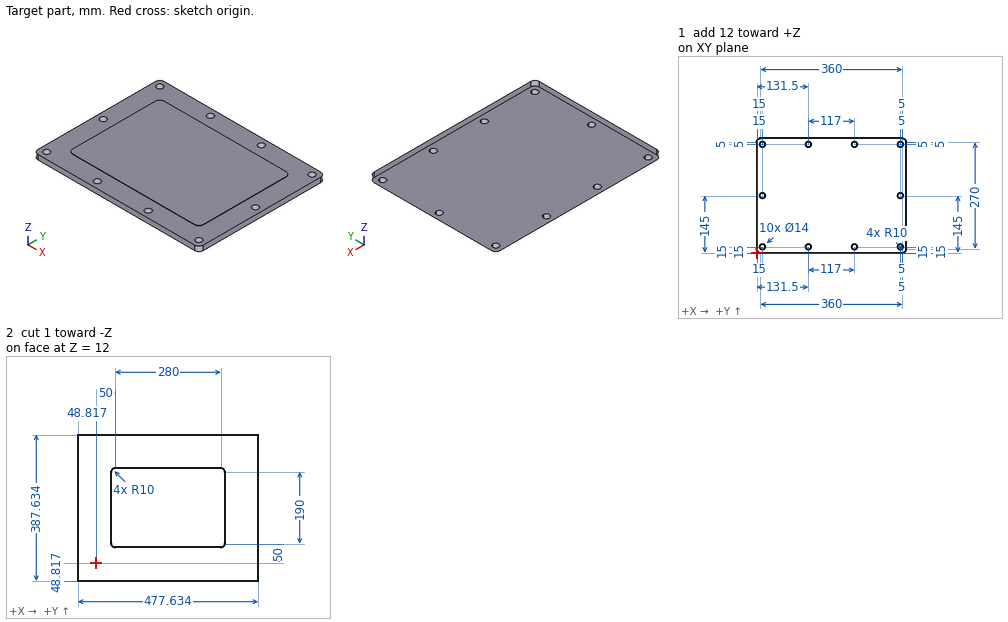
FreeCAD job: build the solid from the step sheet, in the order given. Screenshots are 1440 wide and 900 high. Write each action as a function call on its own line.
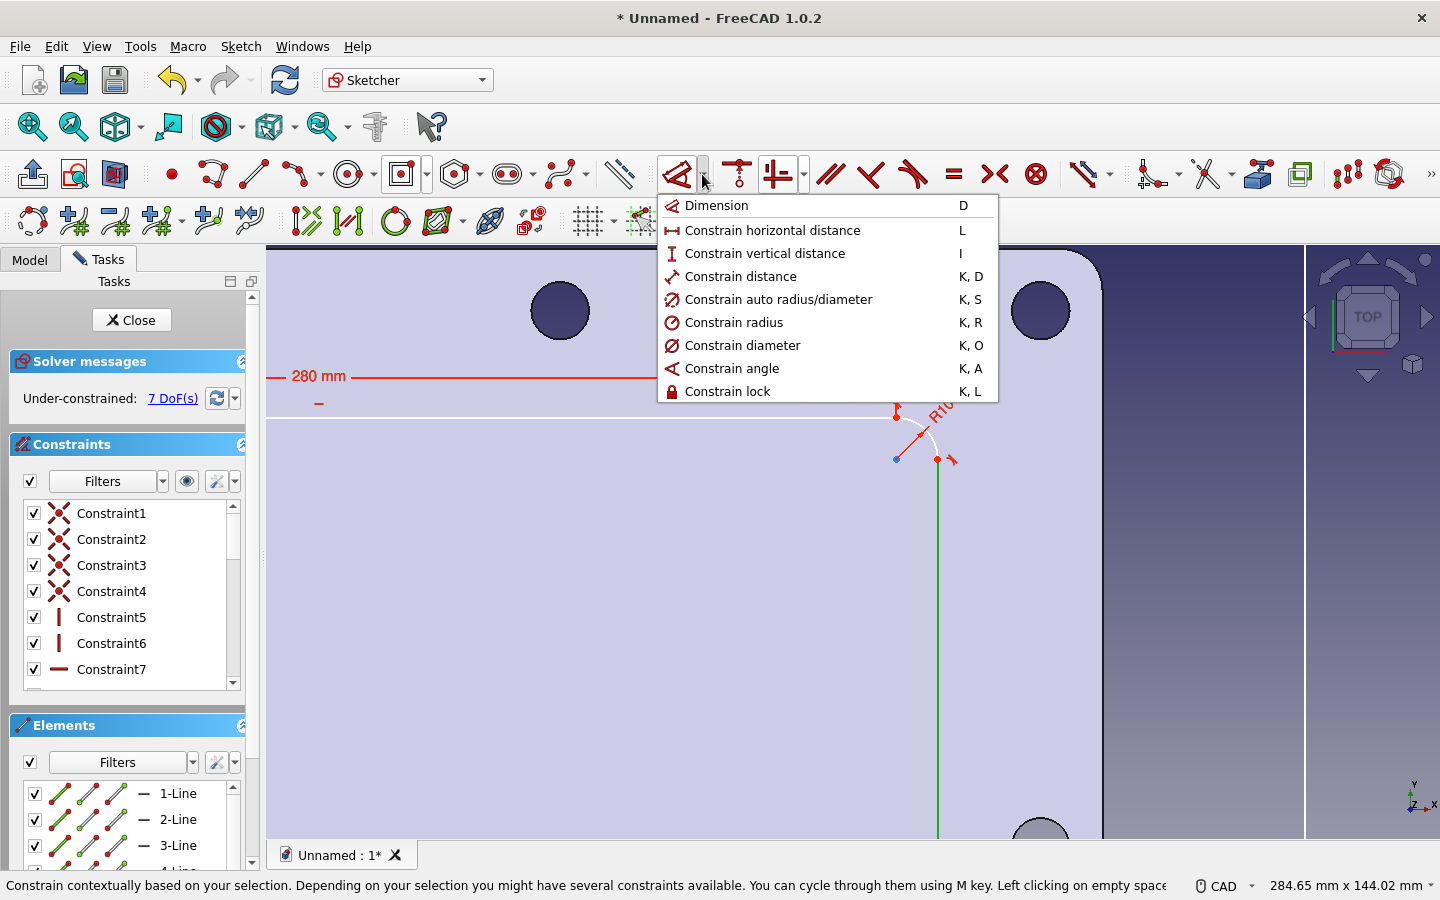
click(828, 254)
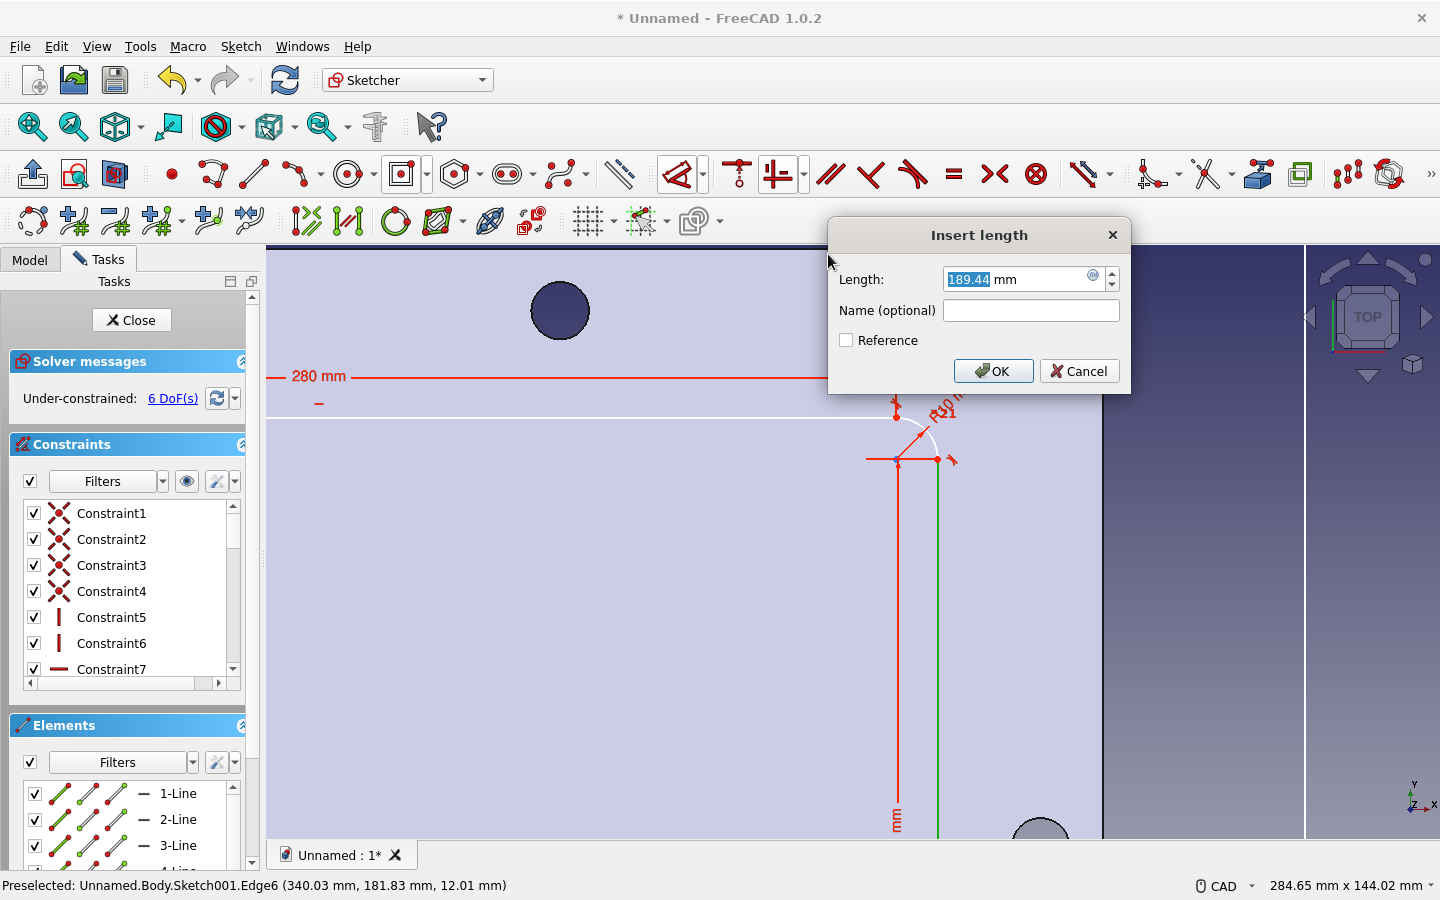
text(190)
key(Return)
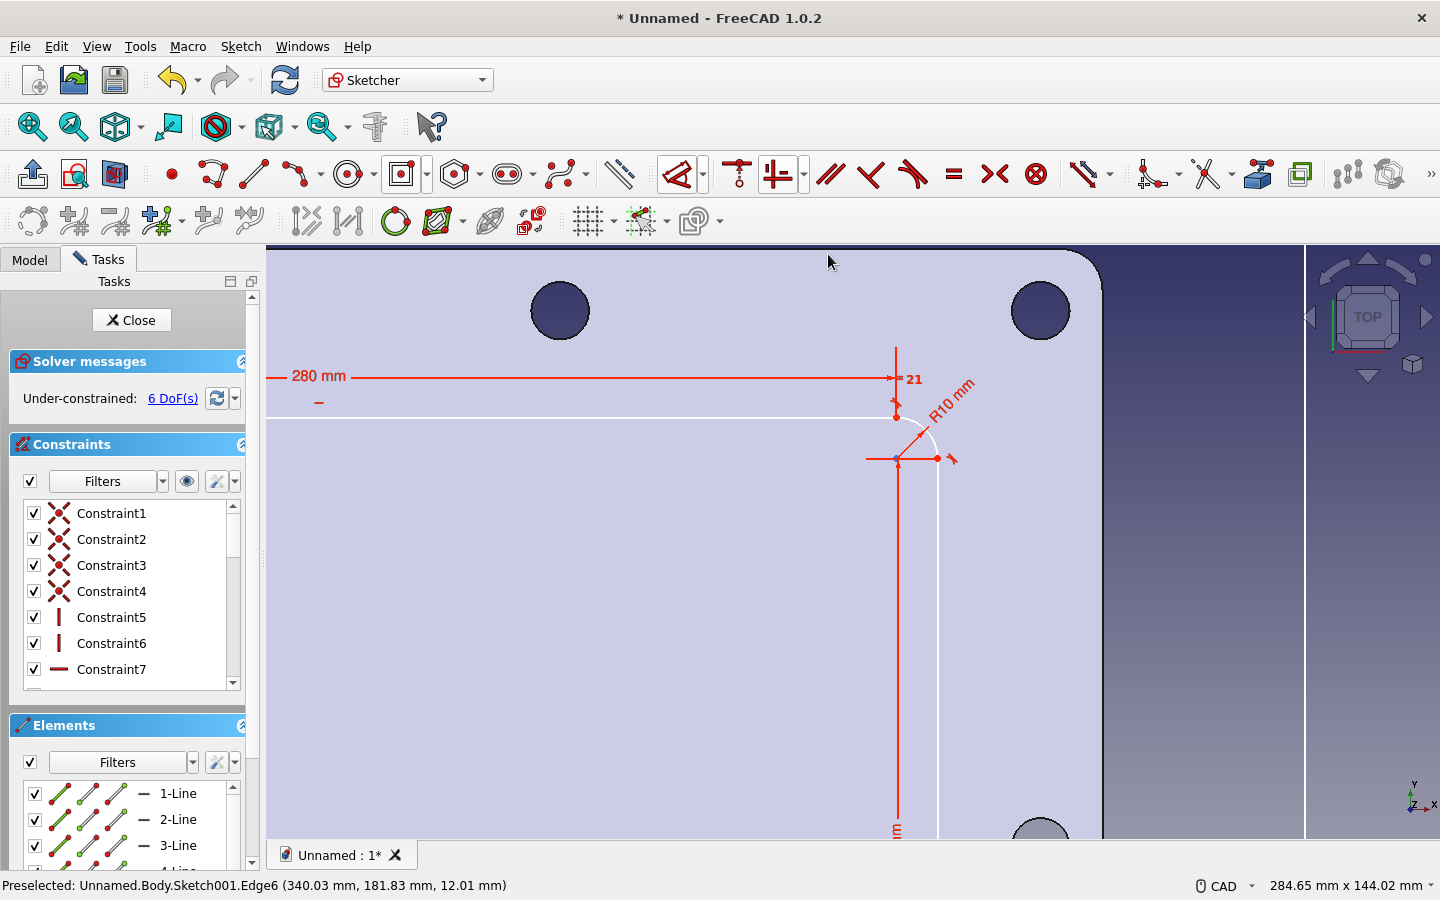
scroll(937, 442, down, 7)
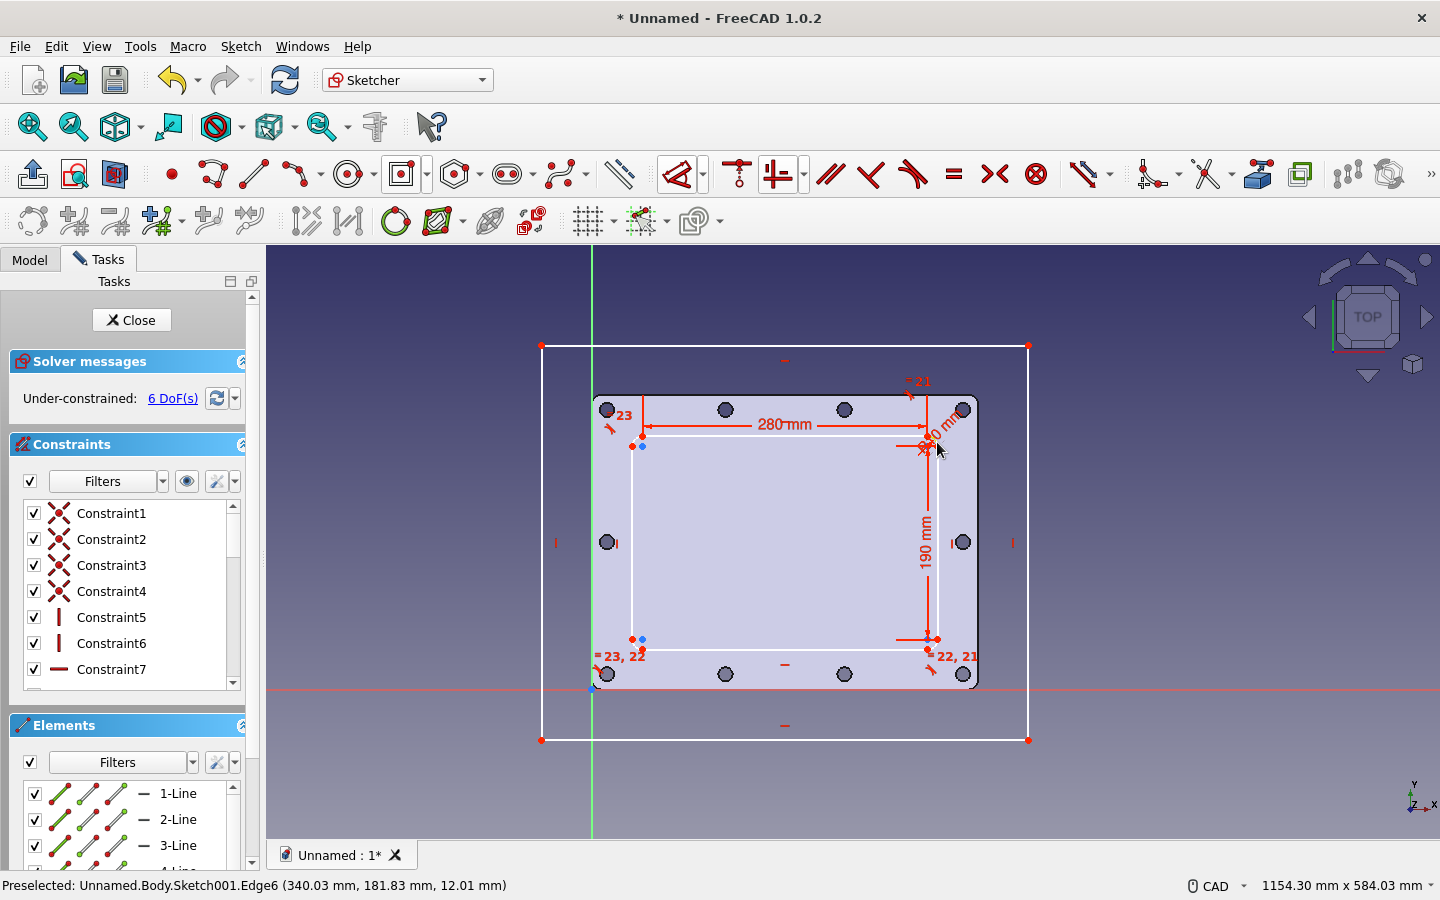
click(643, 436)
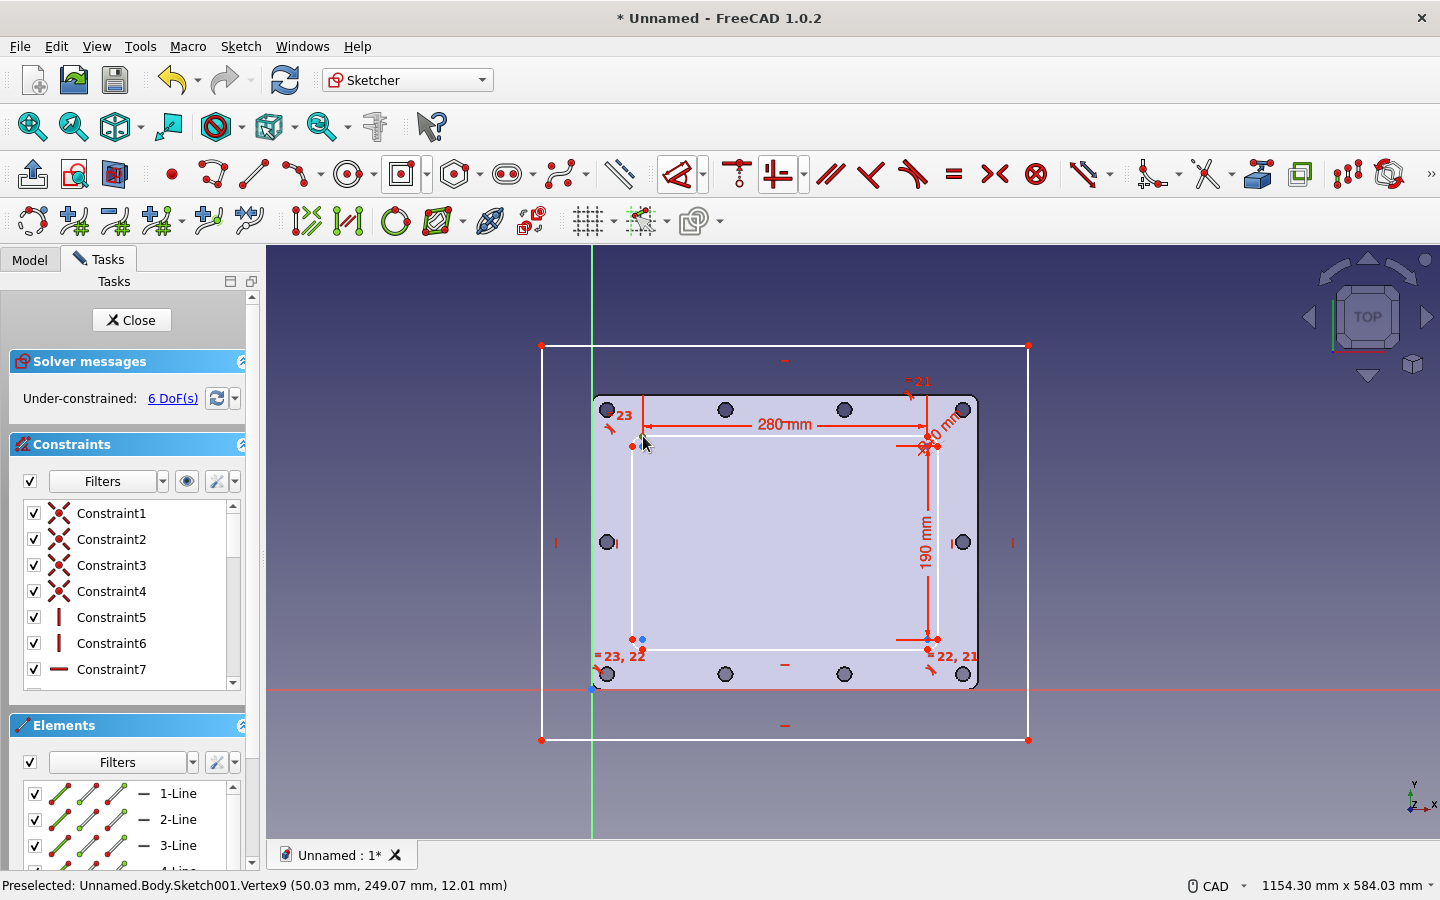
key(l)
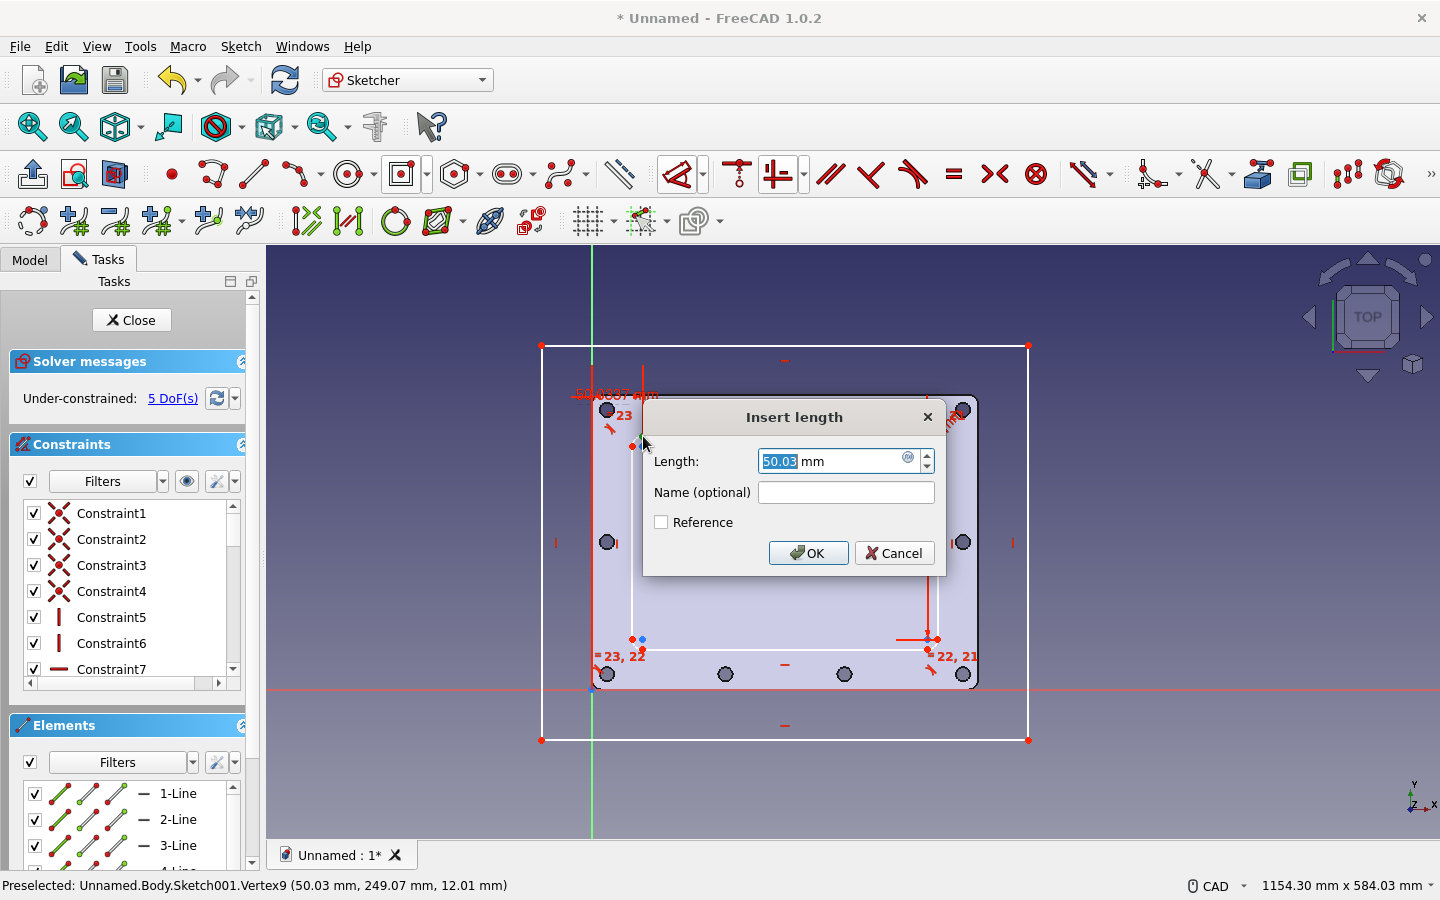
text(50)
key(Return)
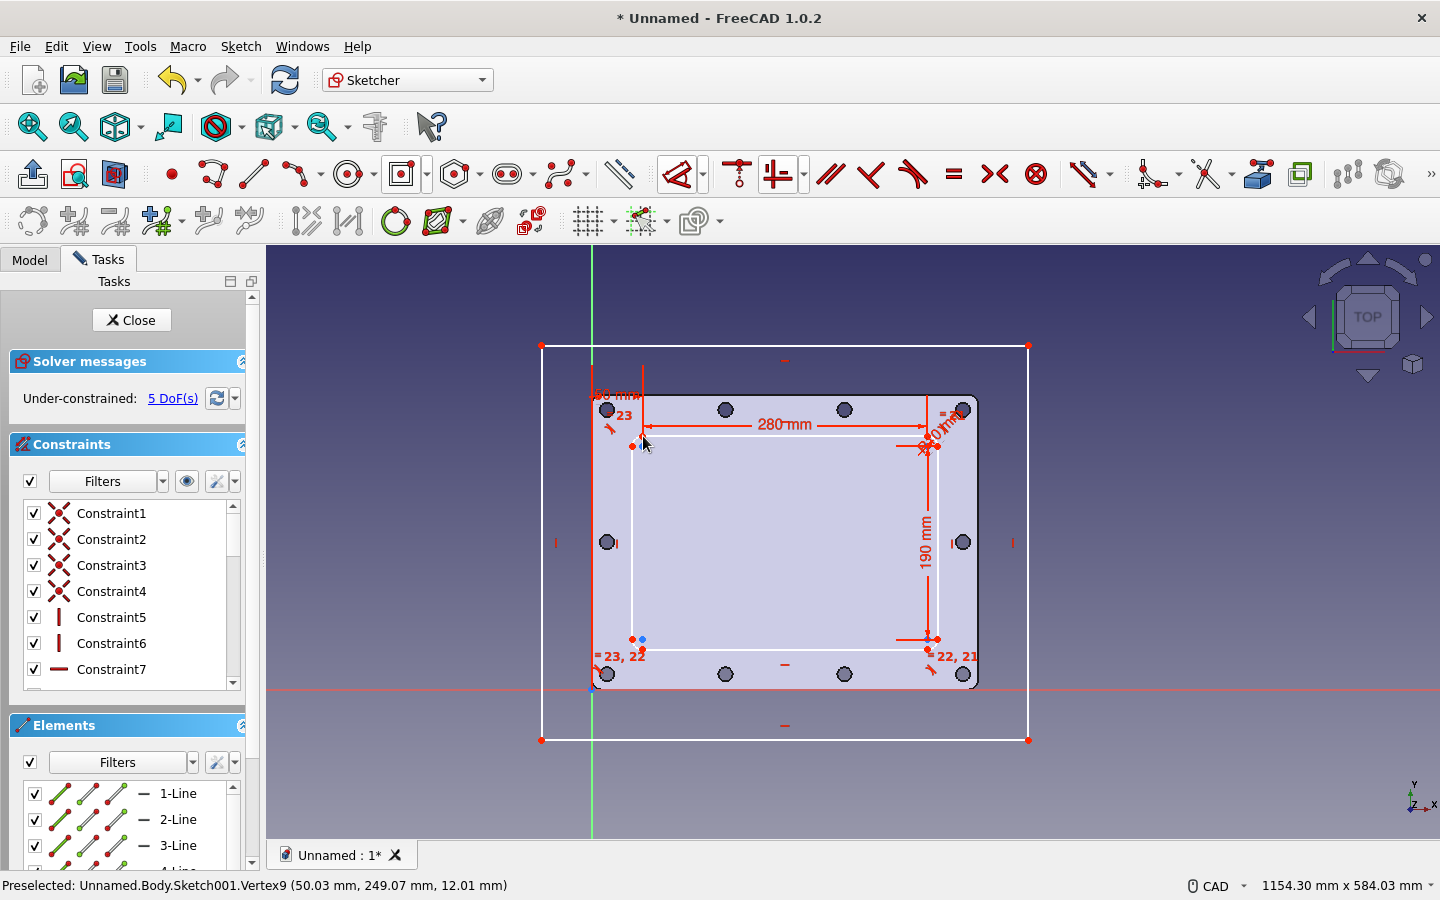
click(938, 640)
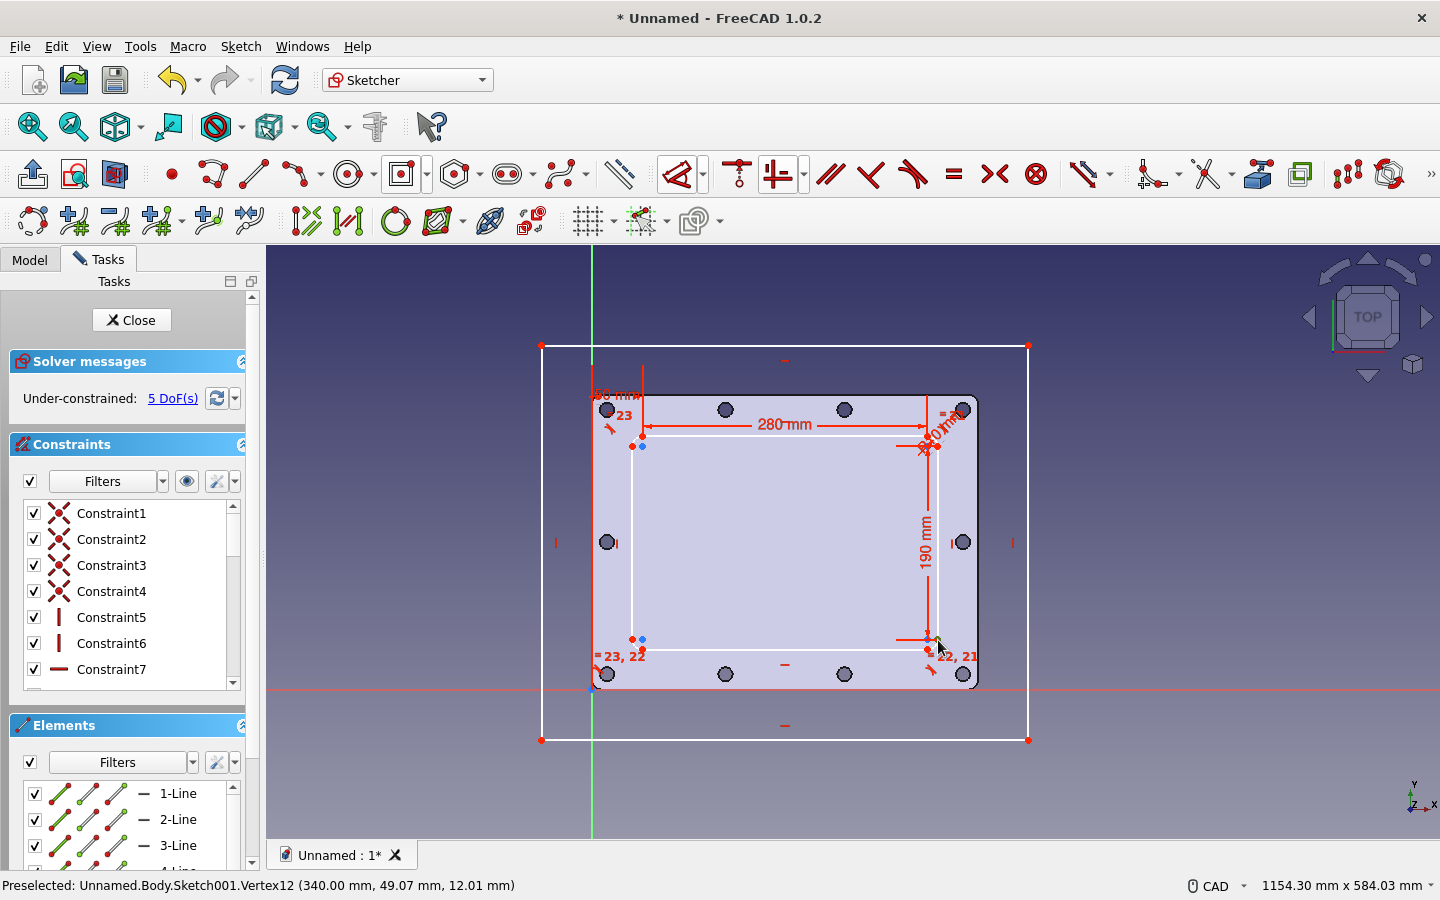
click(702, 174)